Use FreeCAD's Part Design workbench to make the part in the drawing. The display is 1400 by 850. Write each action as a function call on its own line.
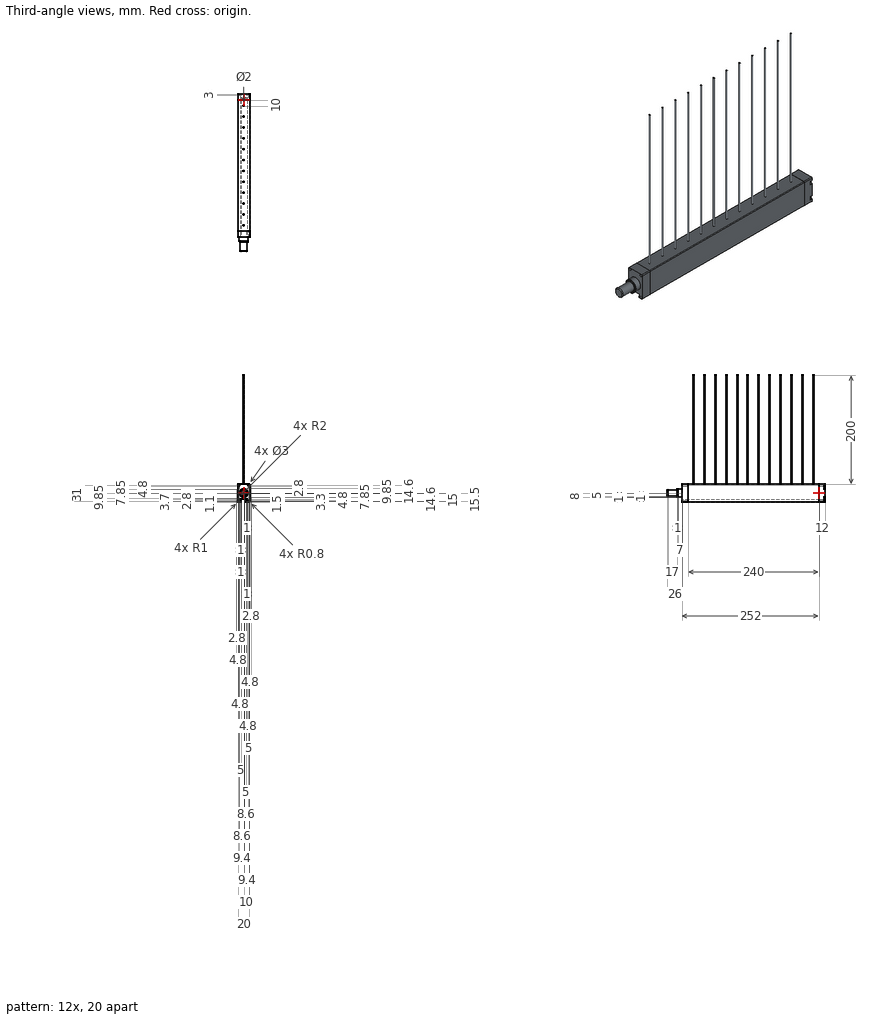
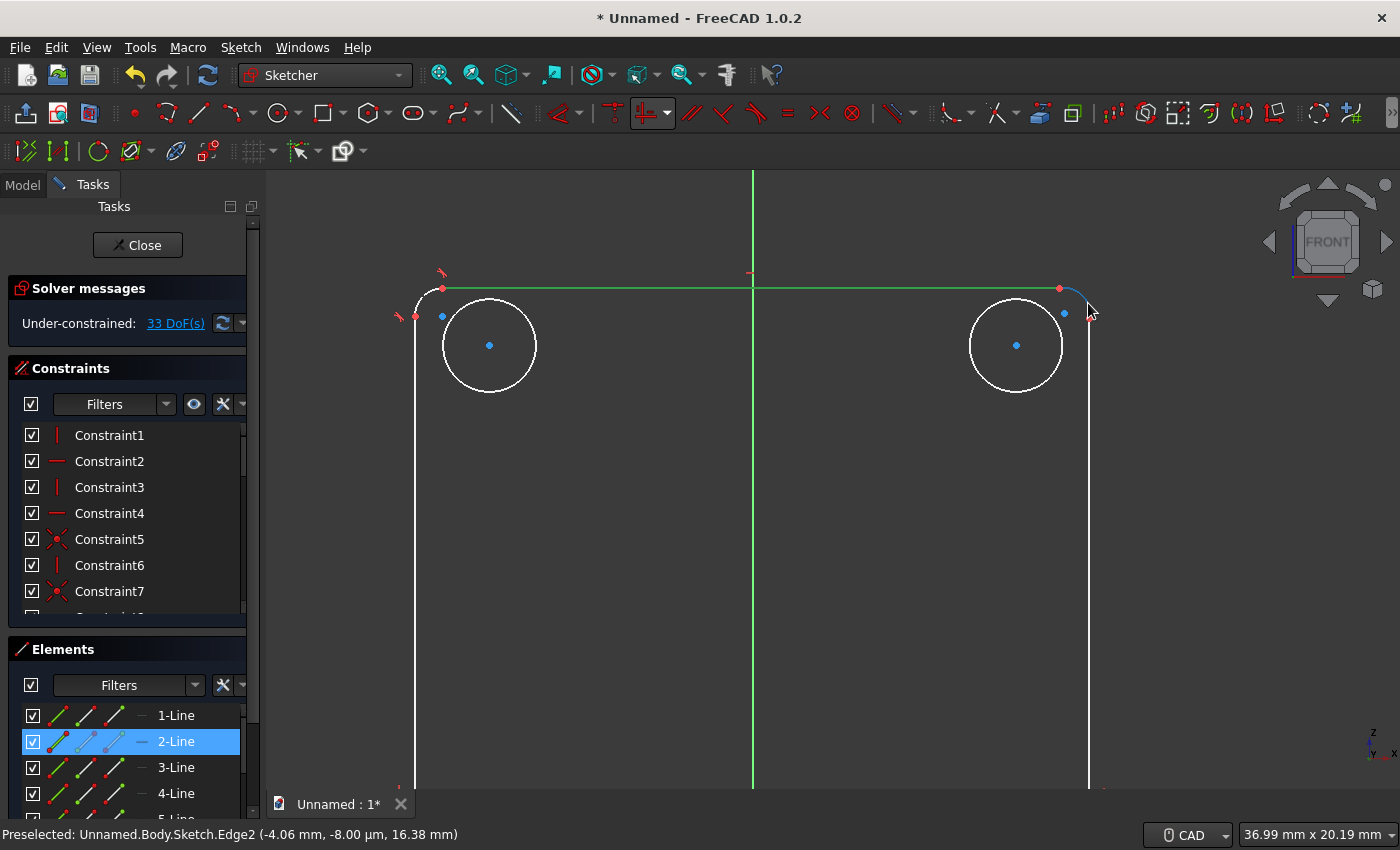
click(1088, 304)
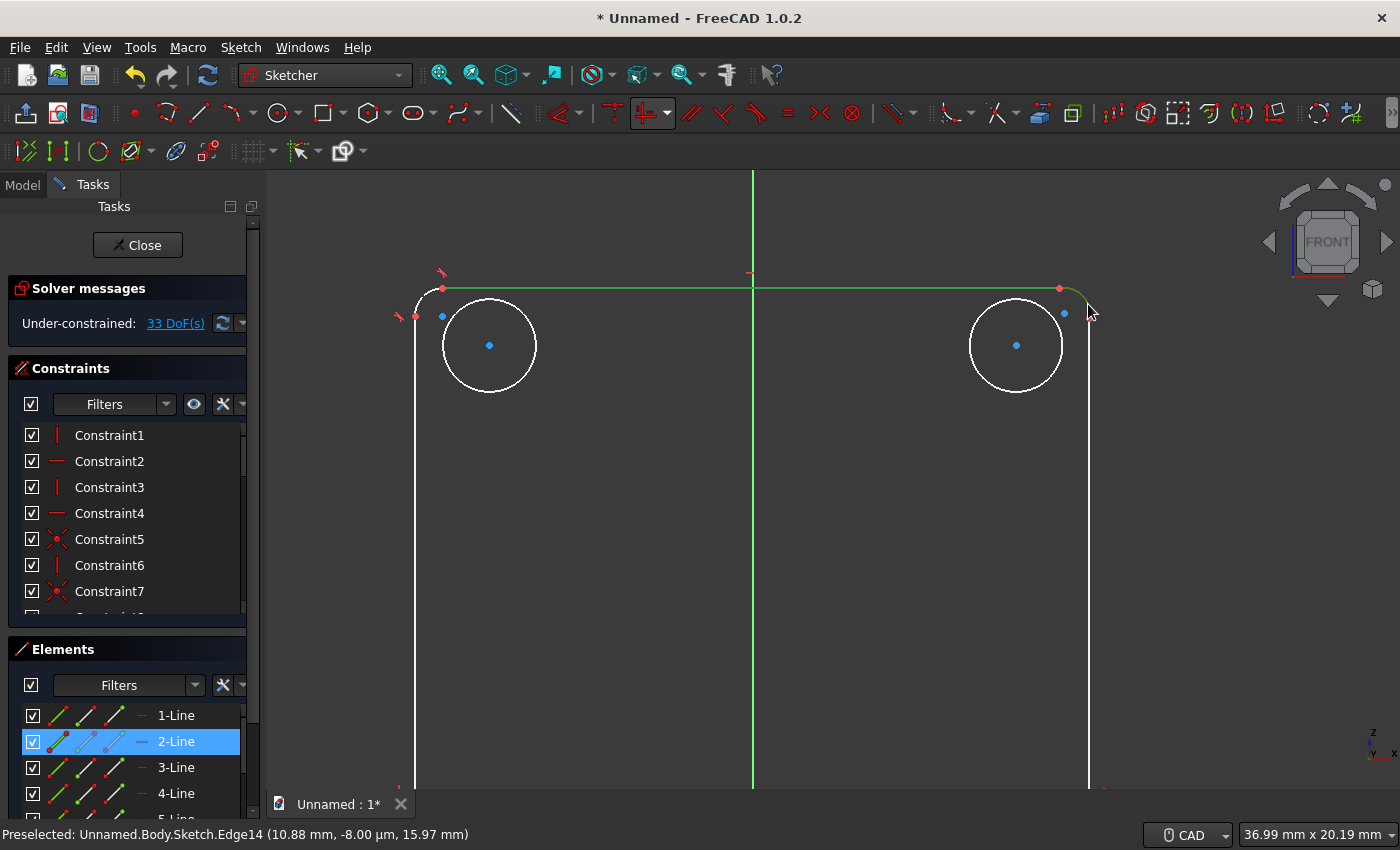
click(756, 114)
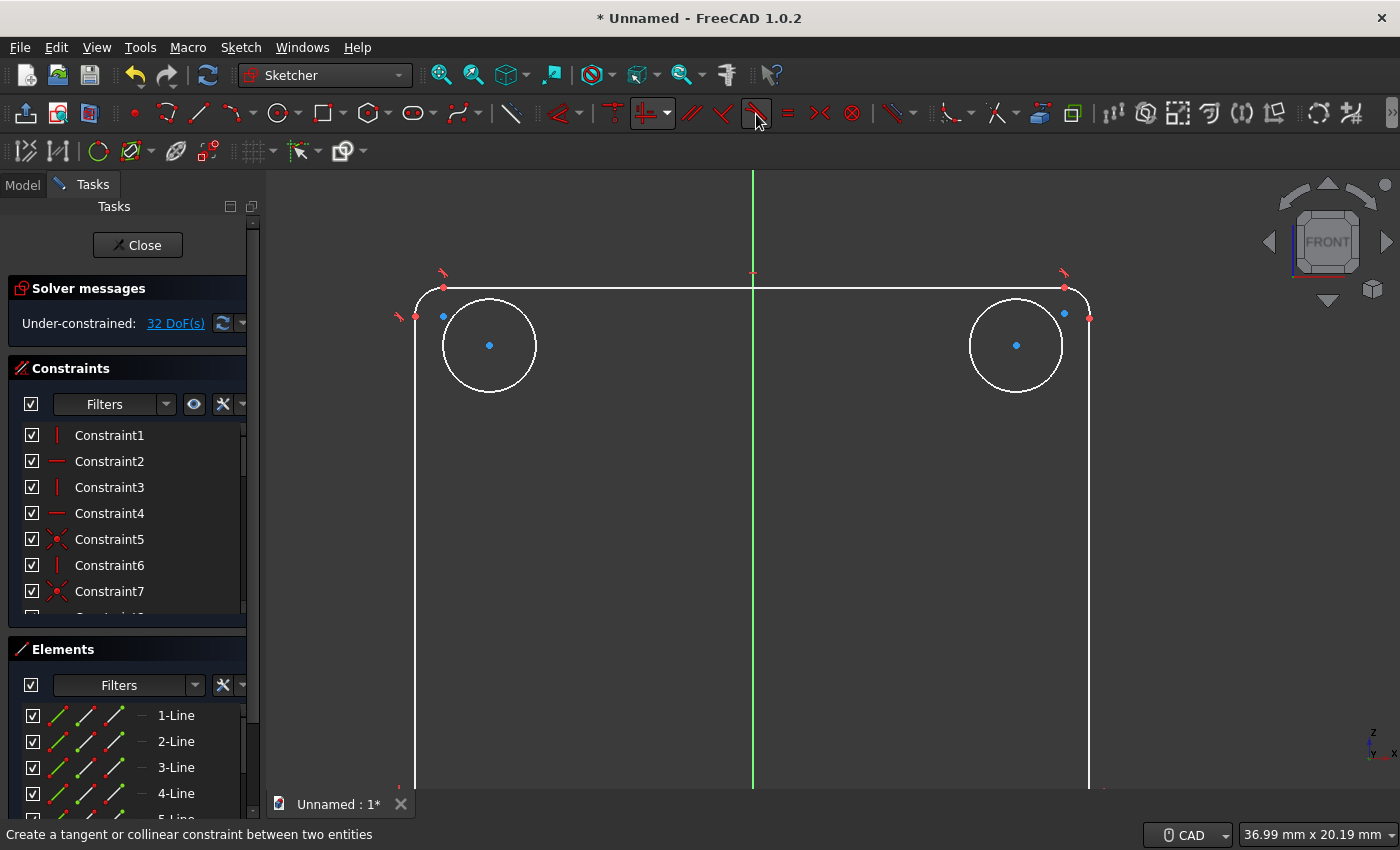
click(1089, 603)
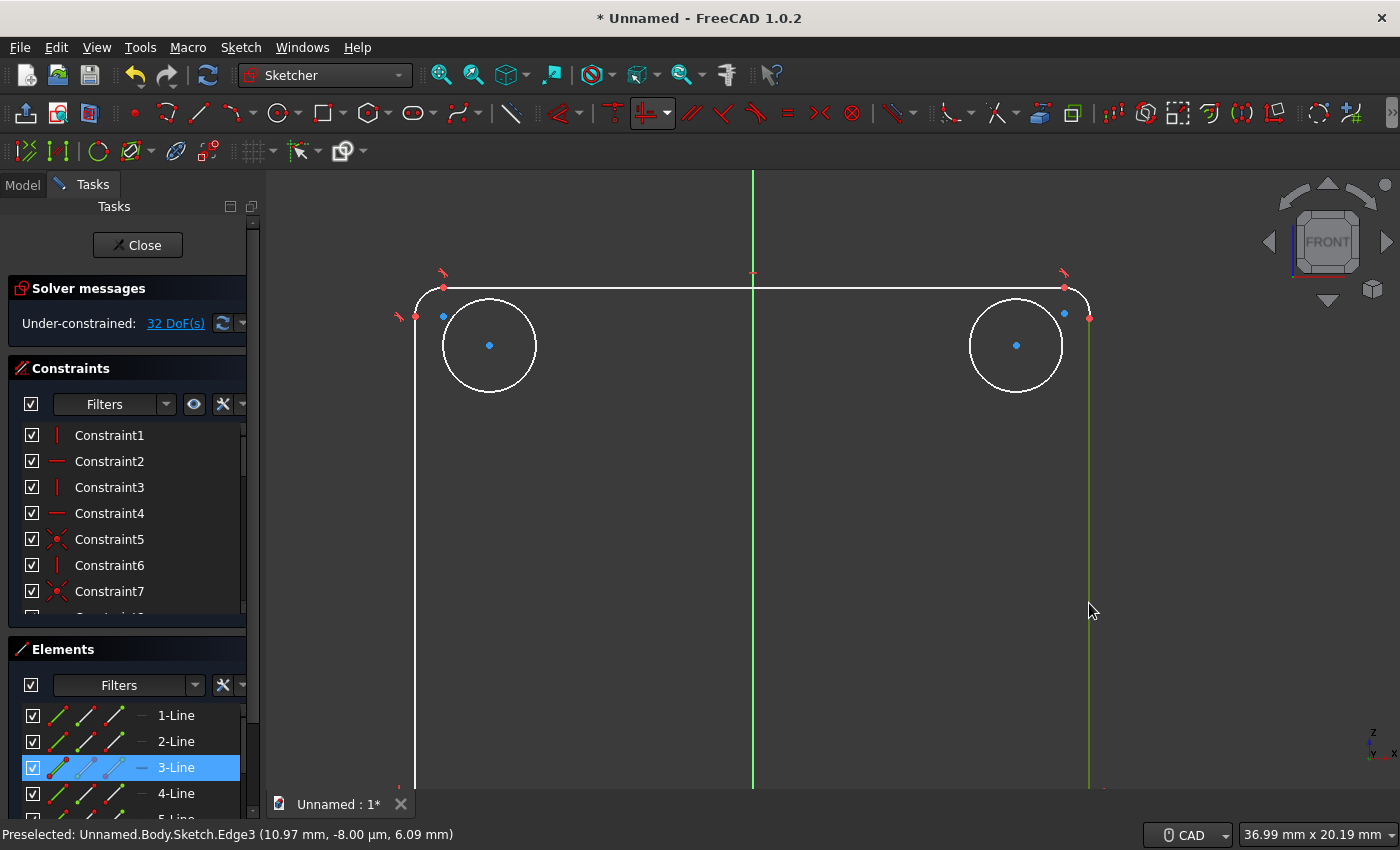
click(1088, 305)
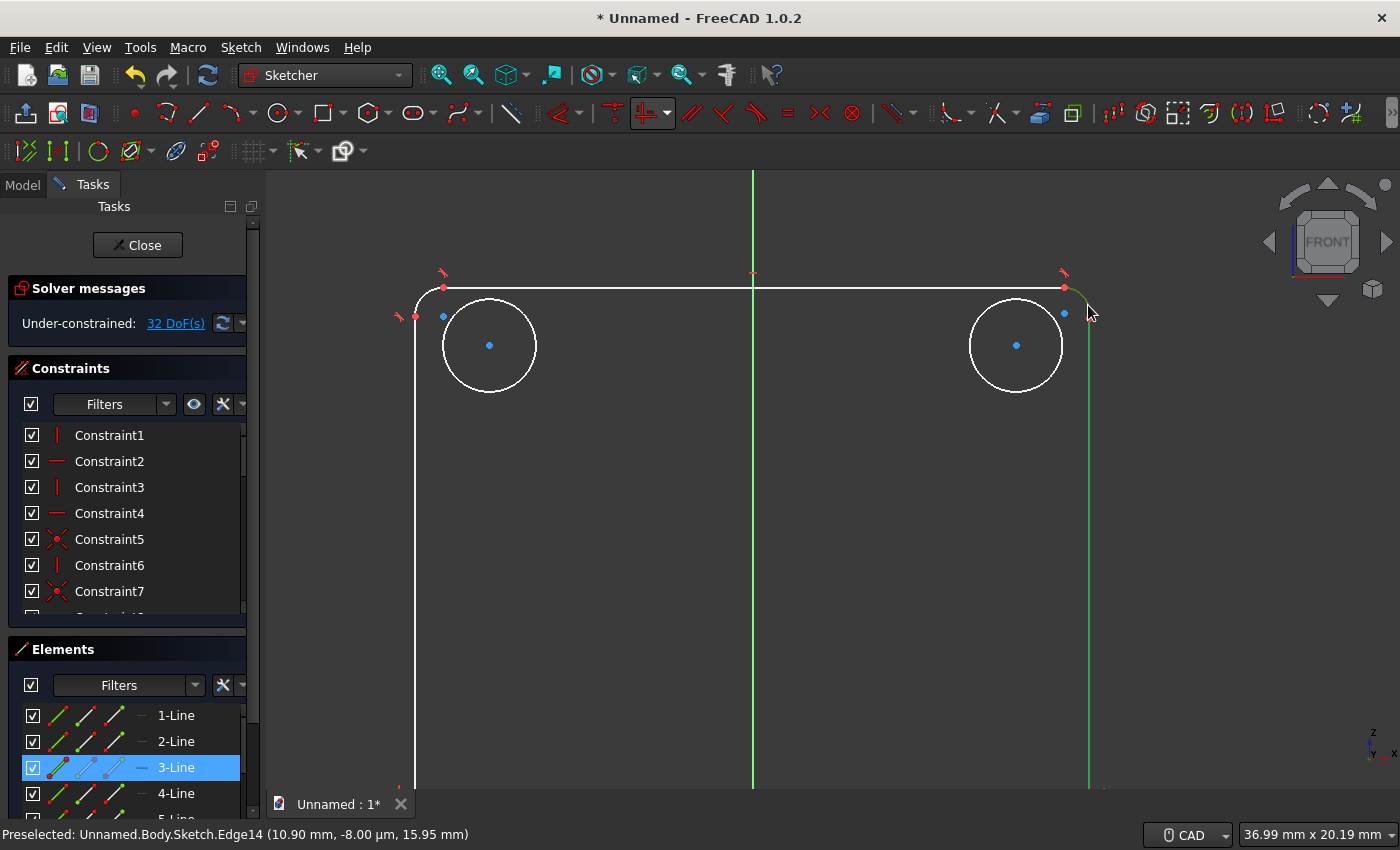
key(t)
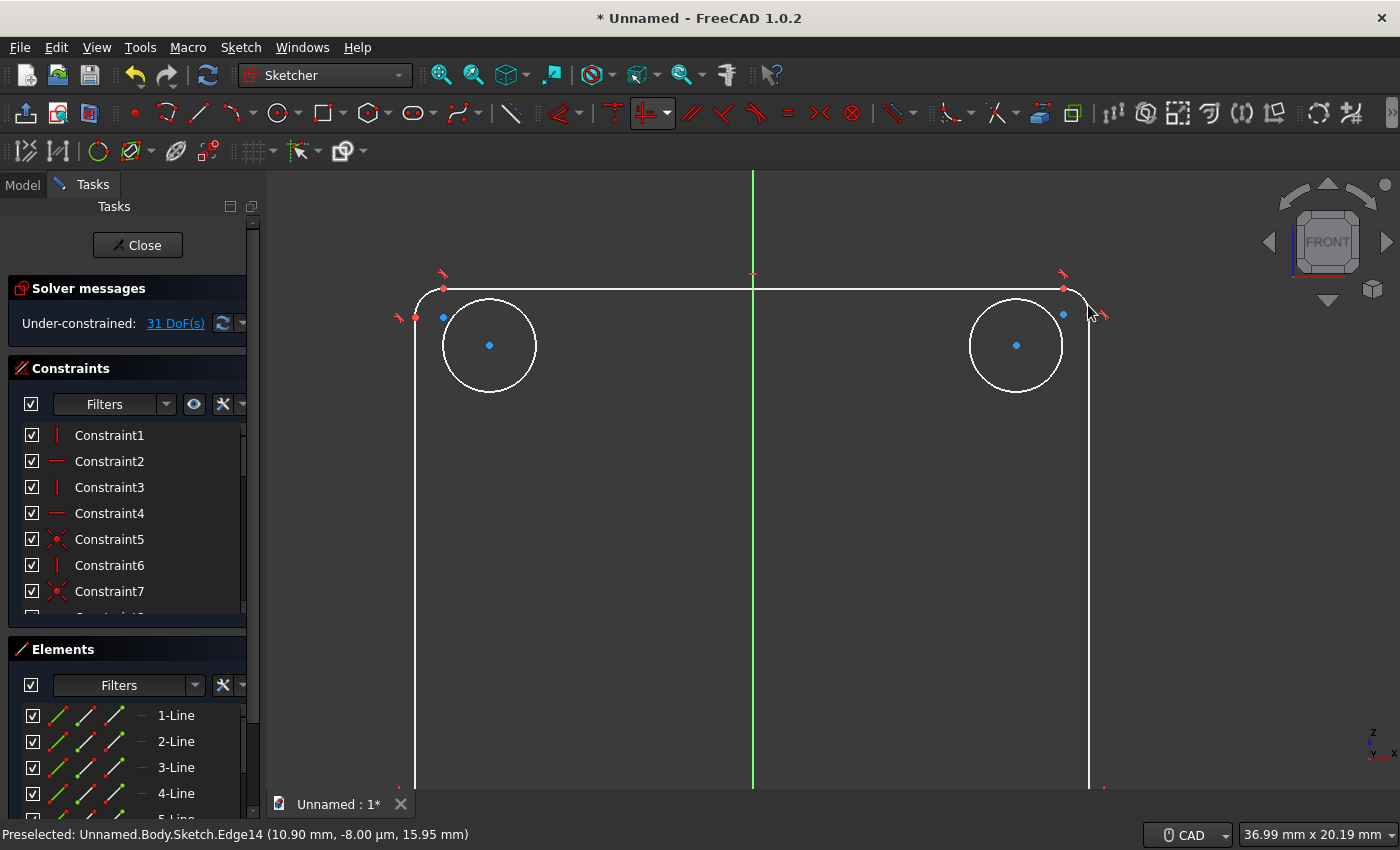
click(1089, 600)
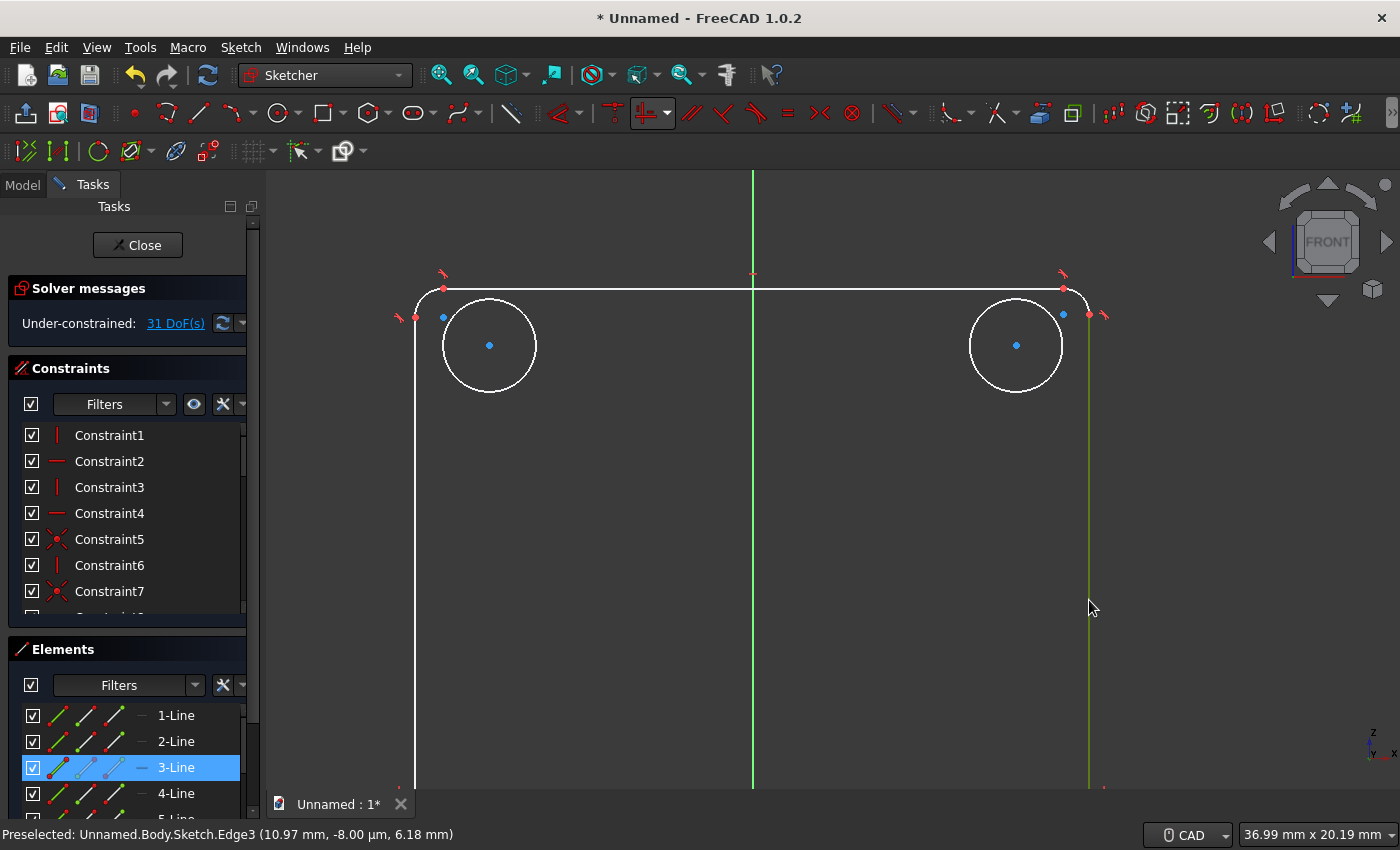
scroll(771, 298, down, 5)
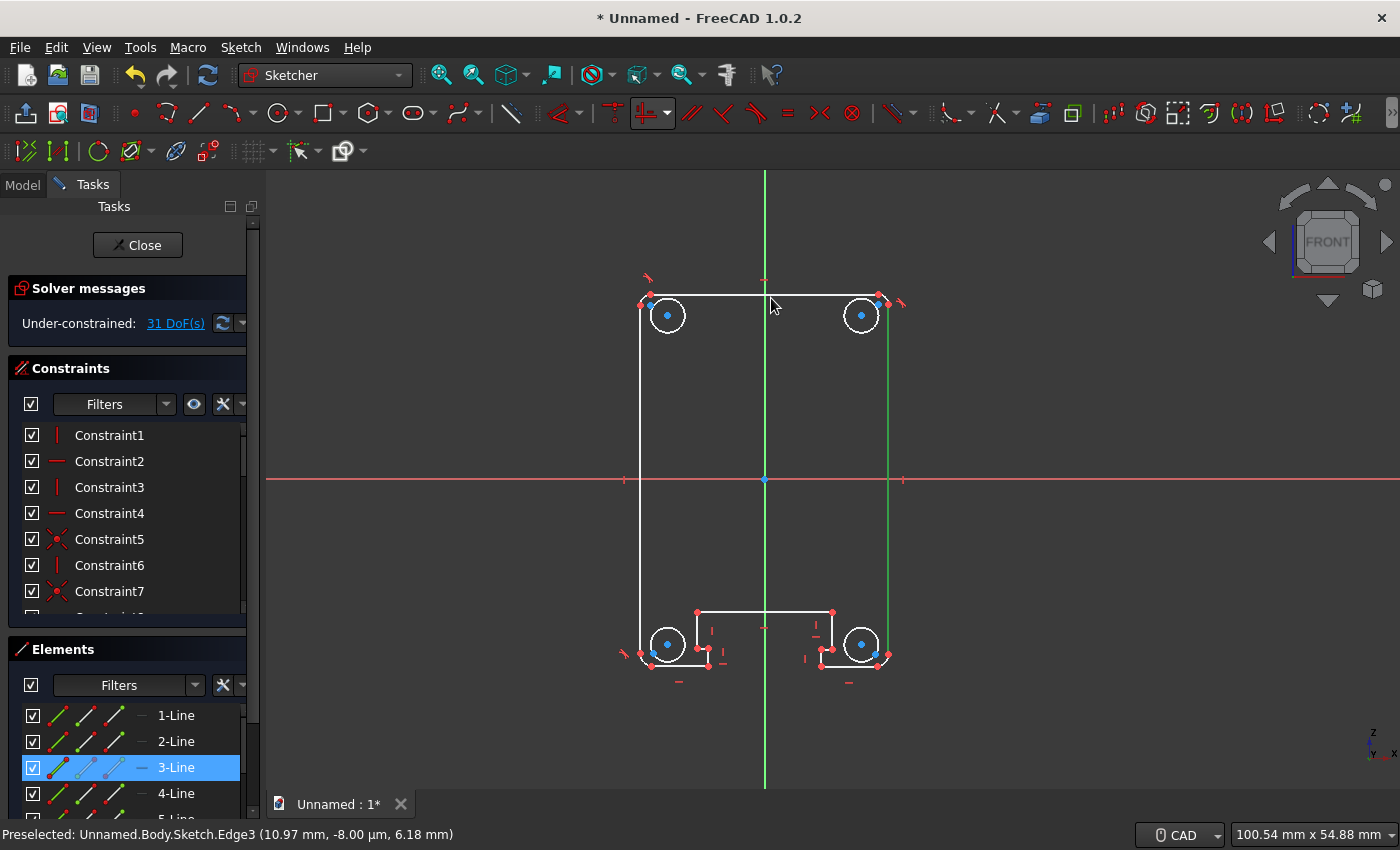
scroll(882, 665, up, 5)